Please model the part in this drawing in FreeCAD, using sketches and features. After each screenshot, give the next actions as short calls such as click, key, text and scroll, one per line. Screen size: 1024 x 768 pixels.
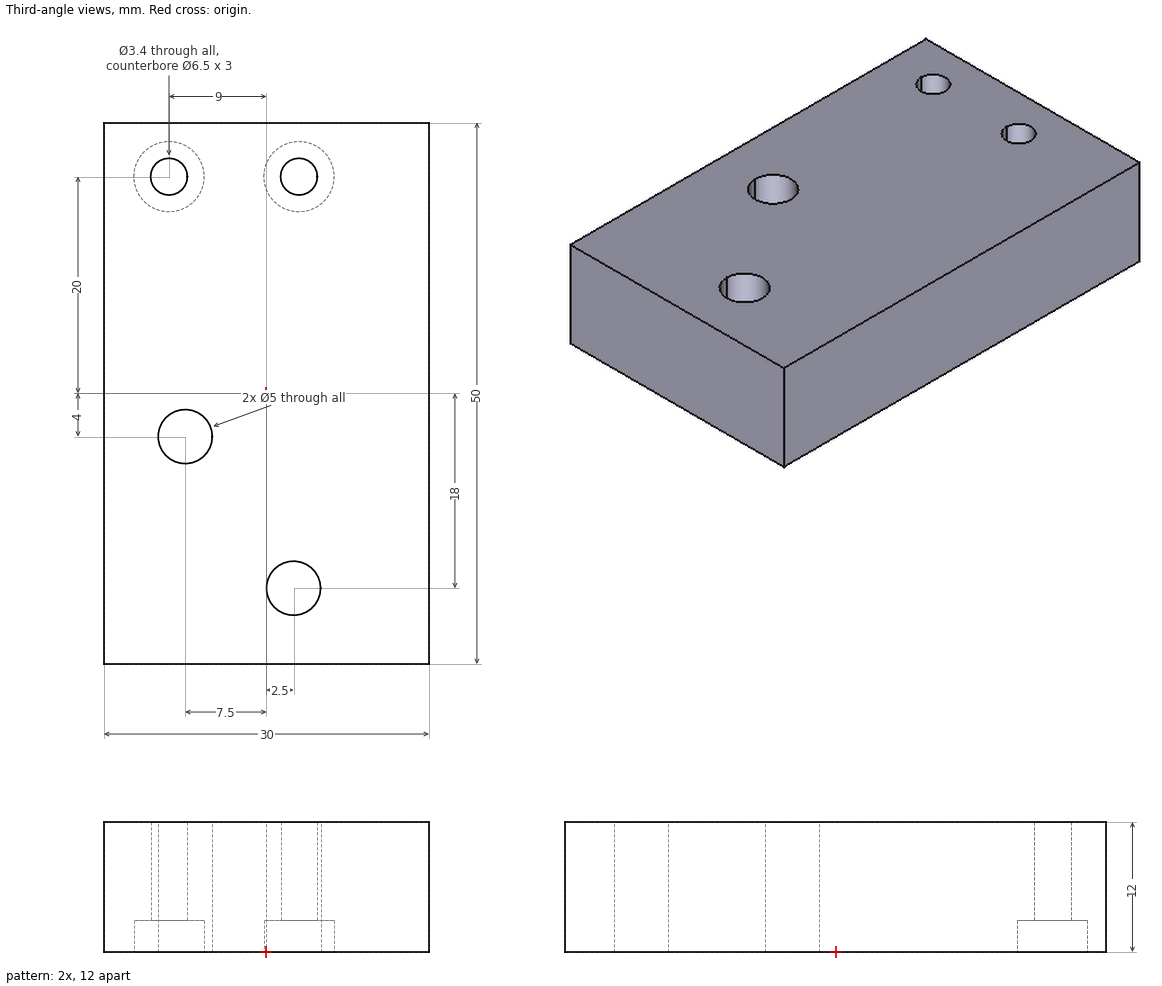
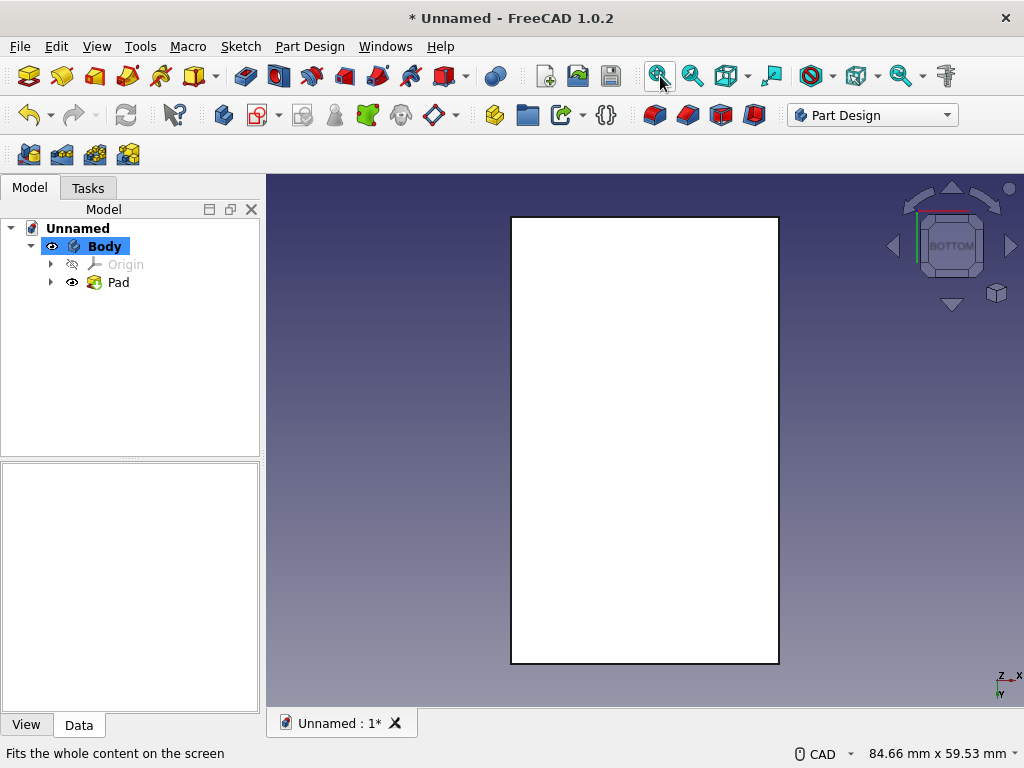
click(645, 503)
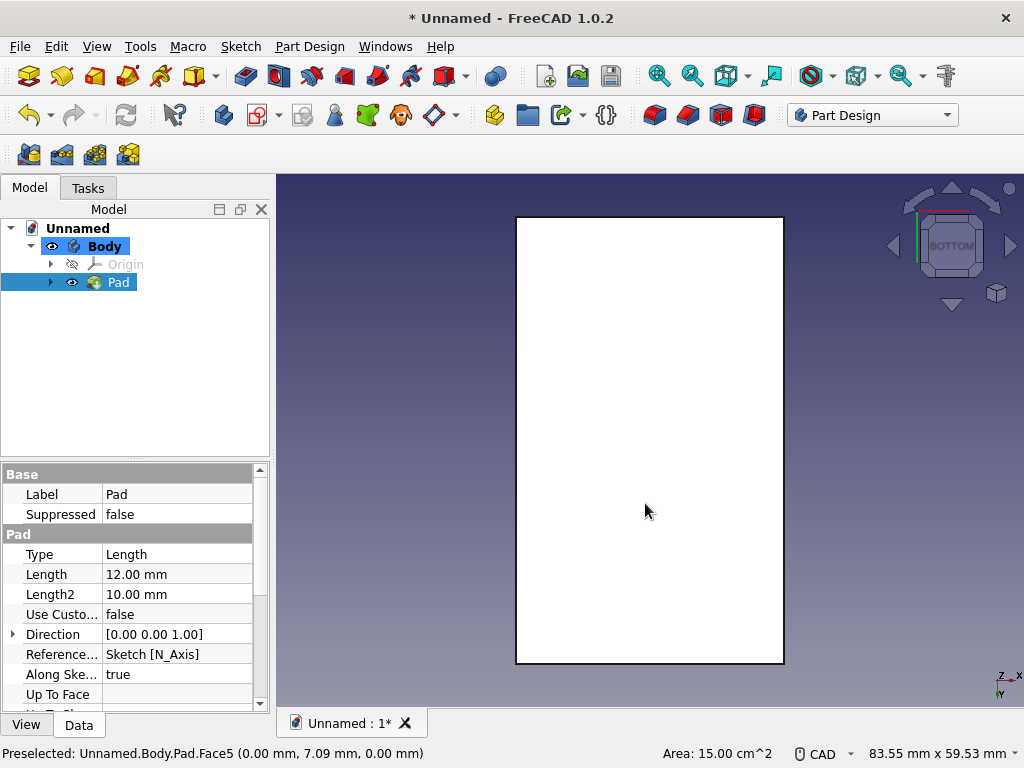
click(256, 116)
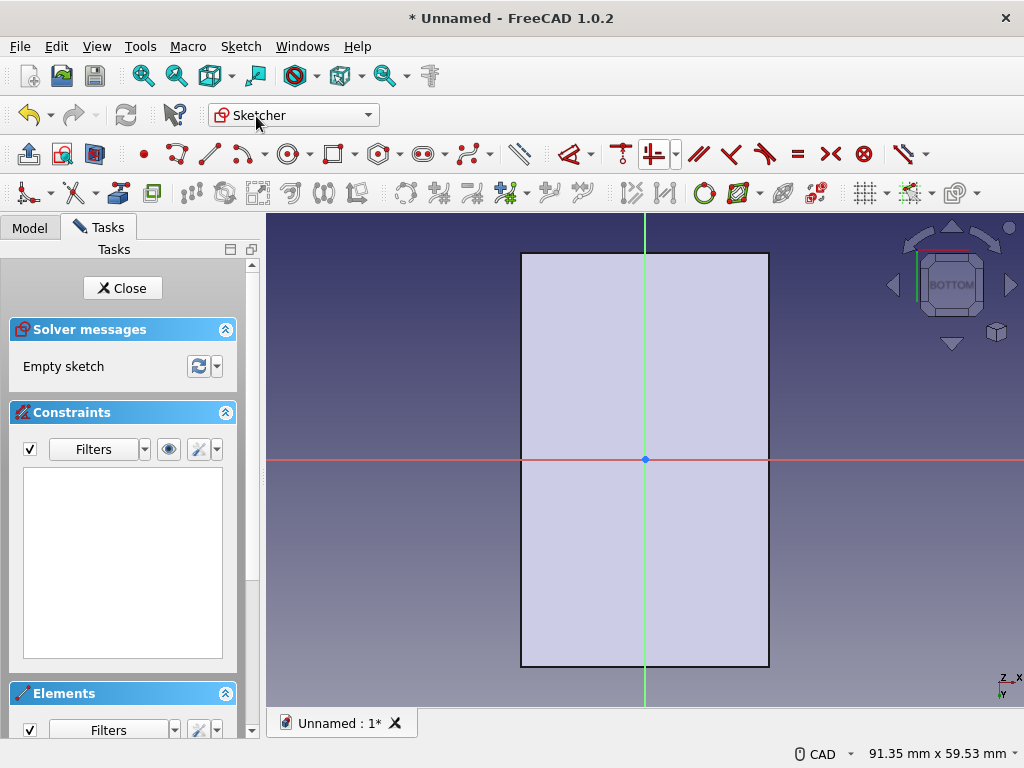
scroll(682, 271, up, 3)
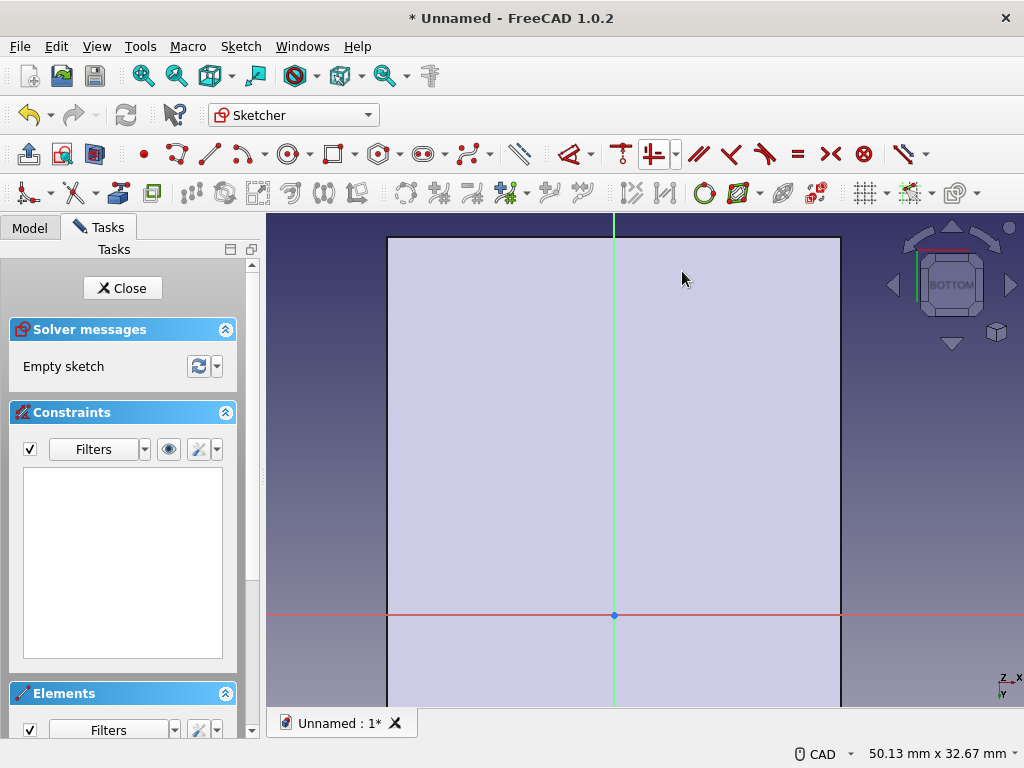
click(288, 154)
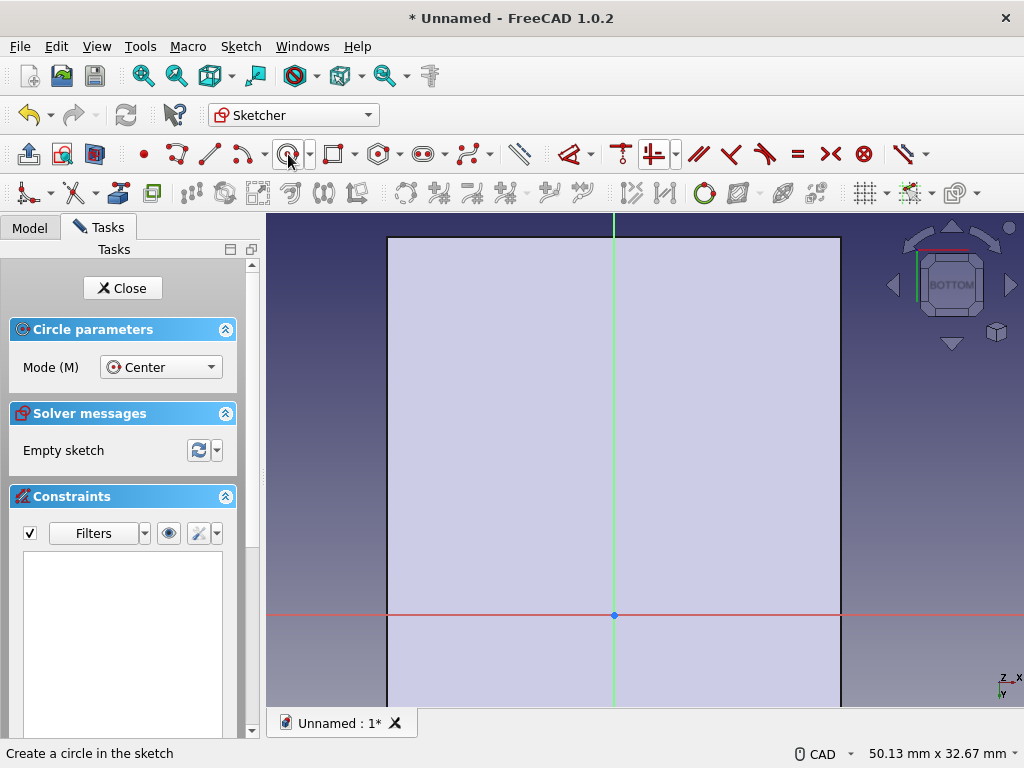
click(501, 555)
move(527, 528)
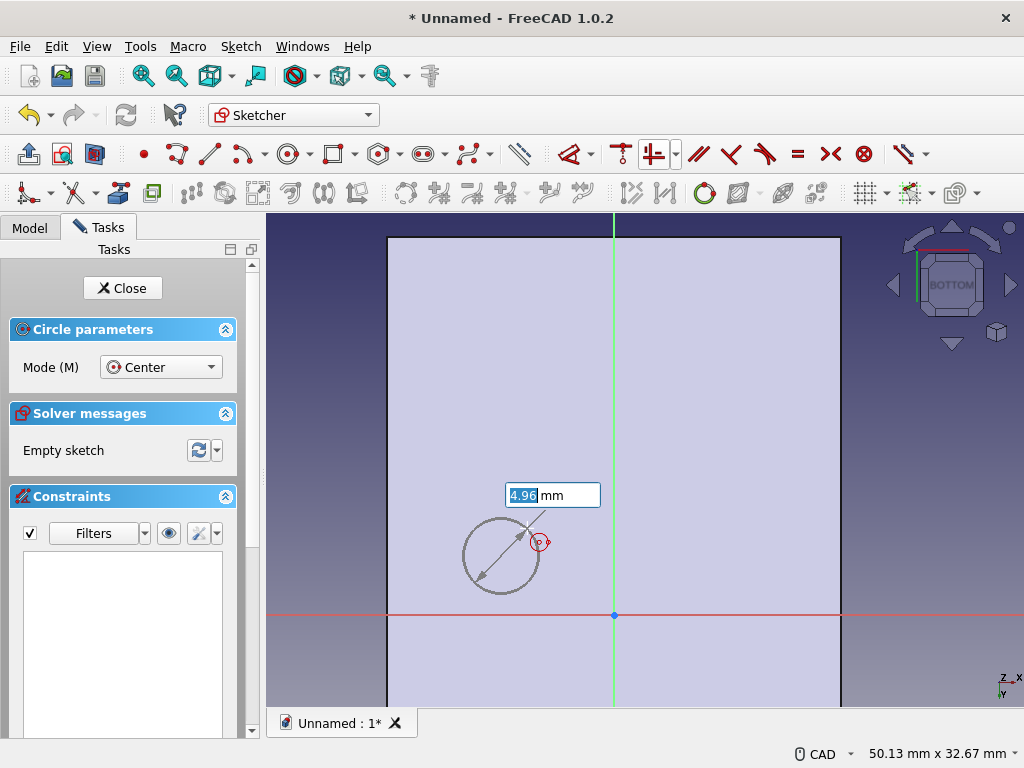
text(5)
key(Return)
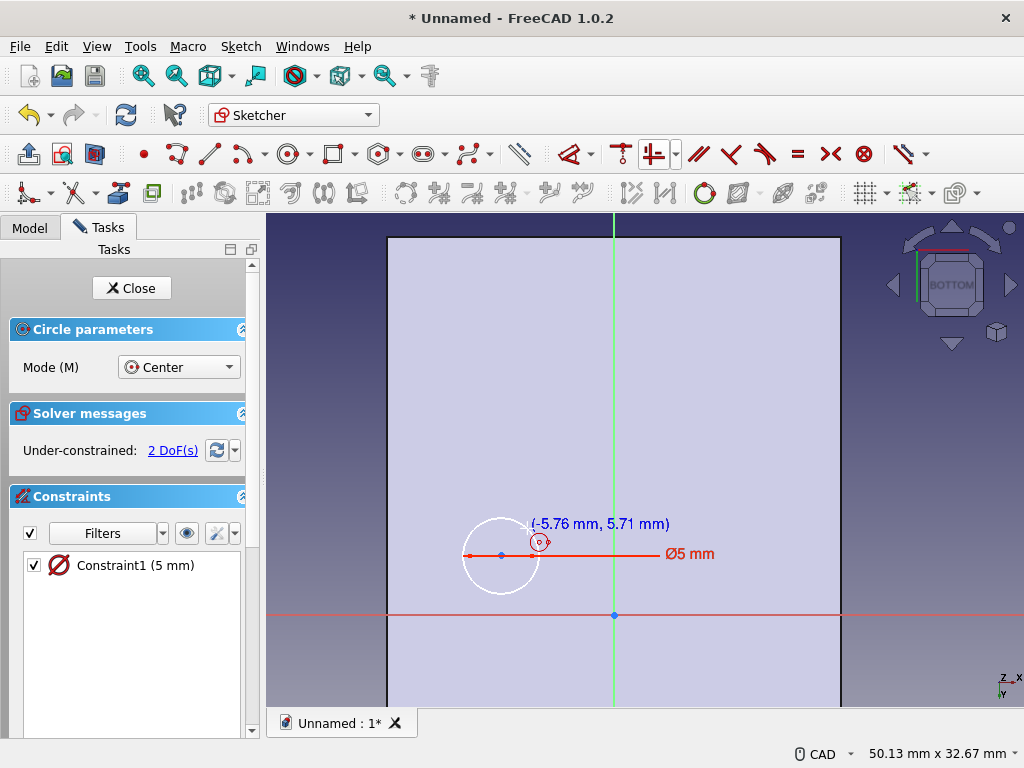
click(652, 343)
move(679, 316)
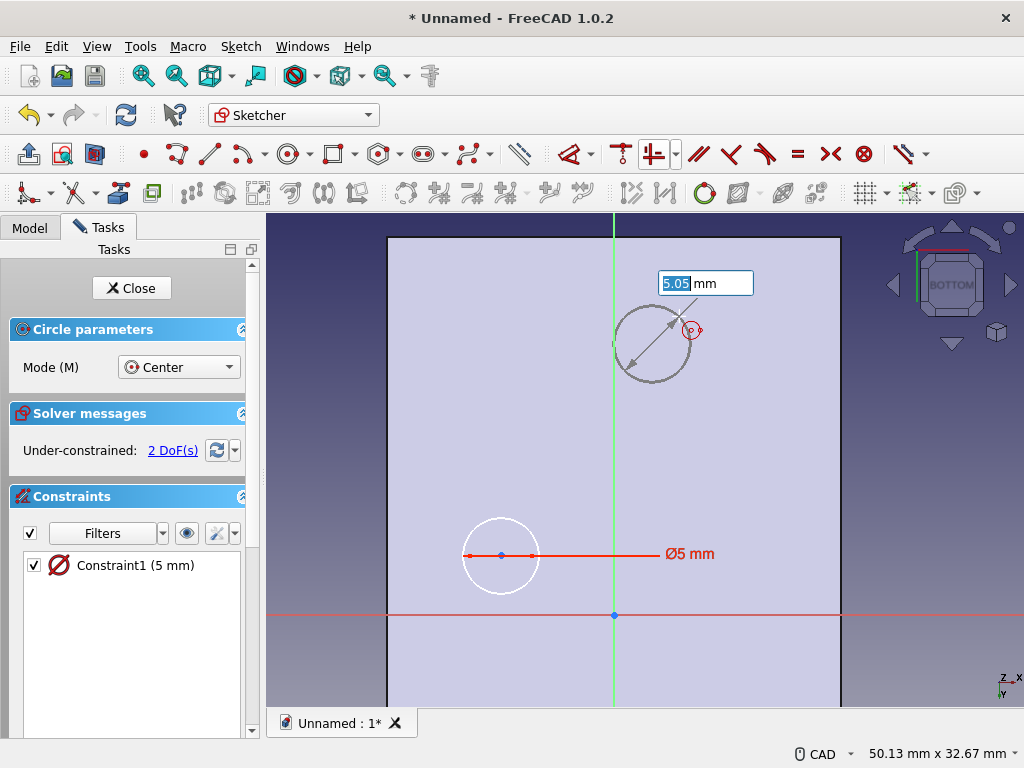
text(5)
key(Return)
key(Escape)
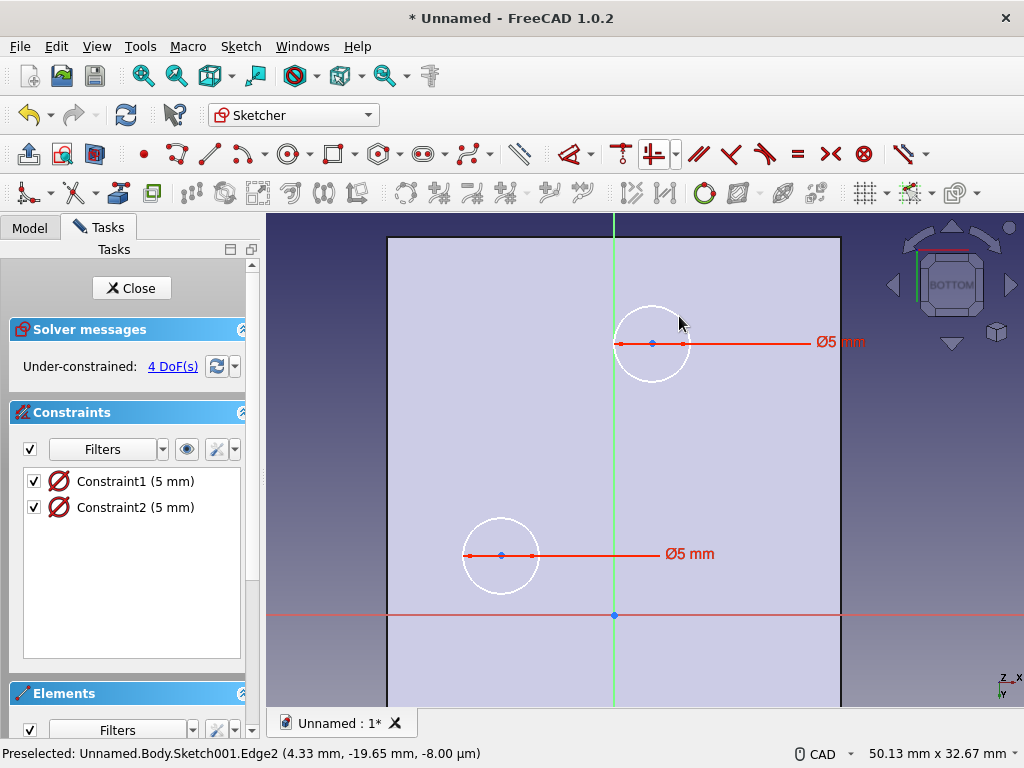
key(d)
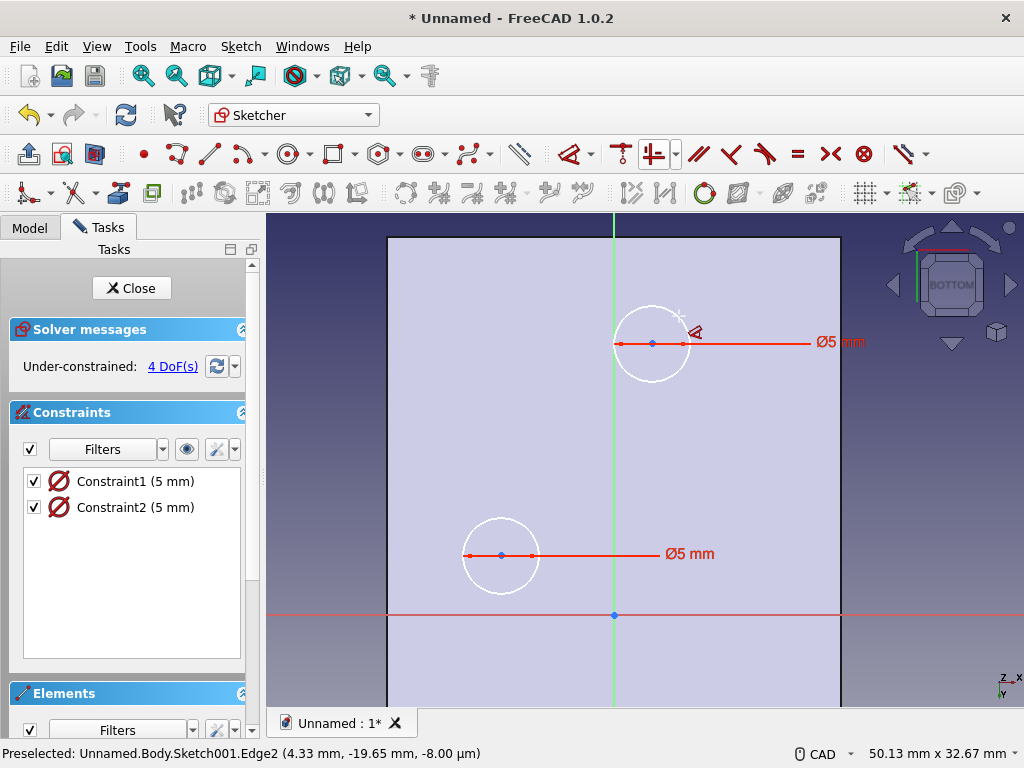
click(501, 556)
click(467, 599)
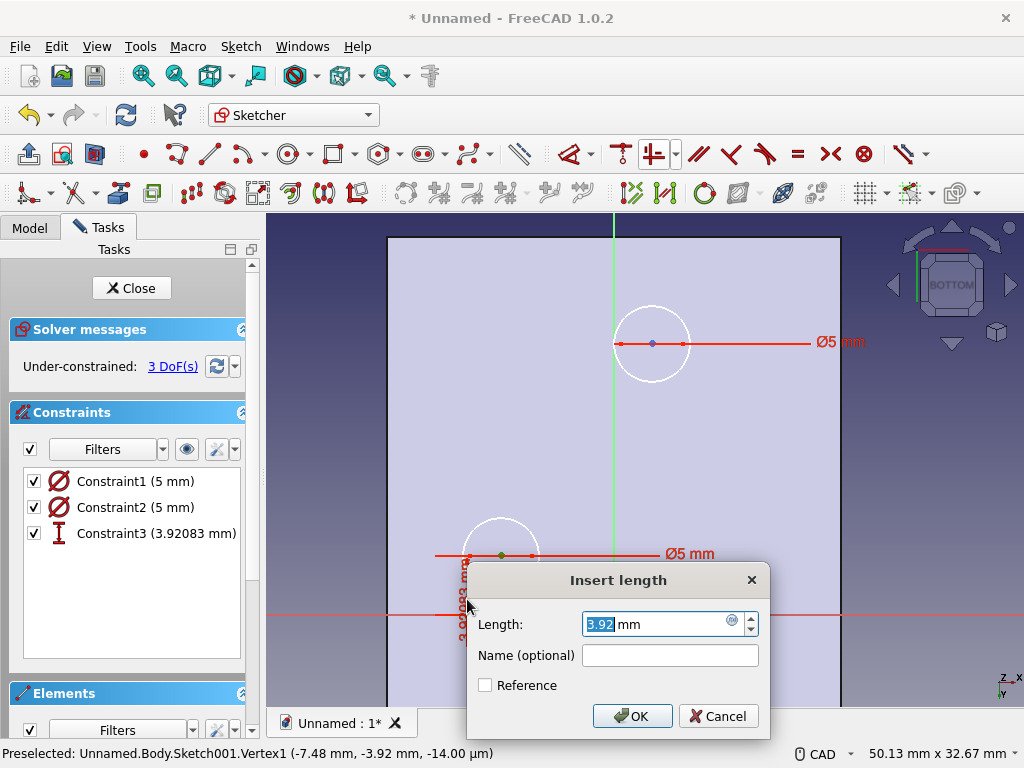
text(4)
key(Return)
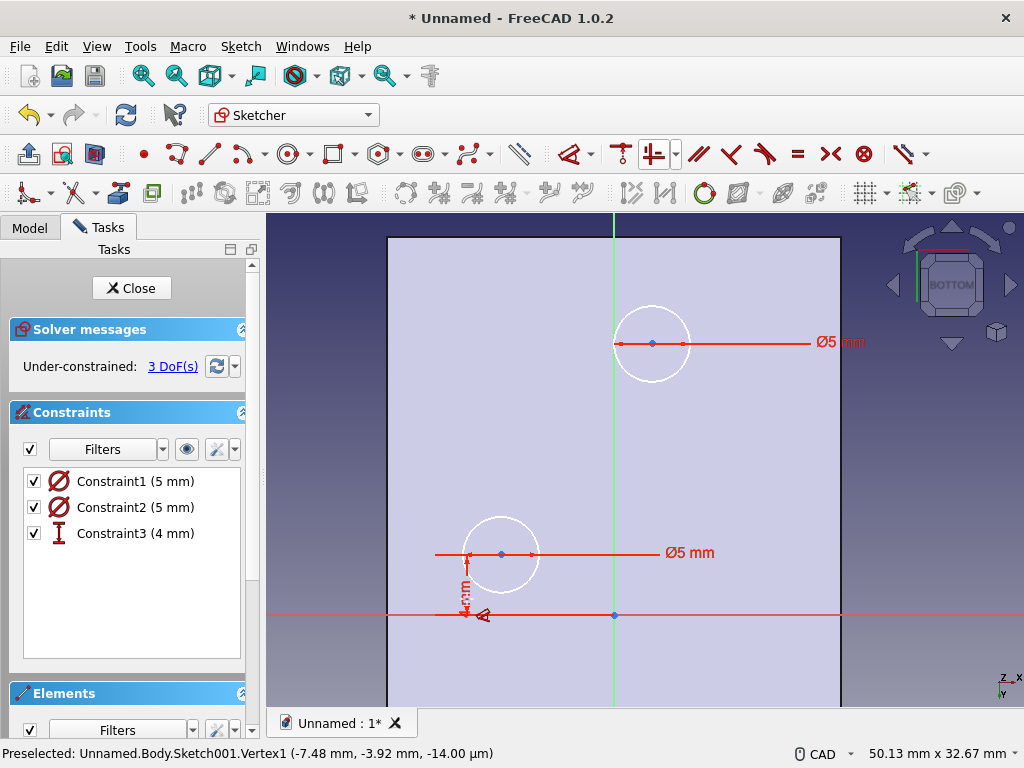
click(652, 344)
click(686, 480)